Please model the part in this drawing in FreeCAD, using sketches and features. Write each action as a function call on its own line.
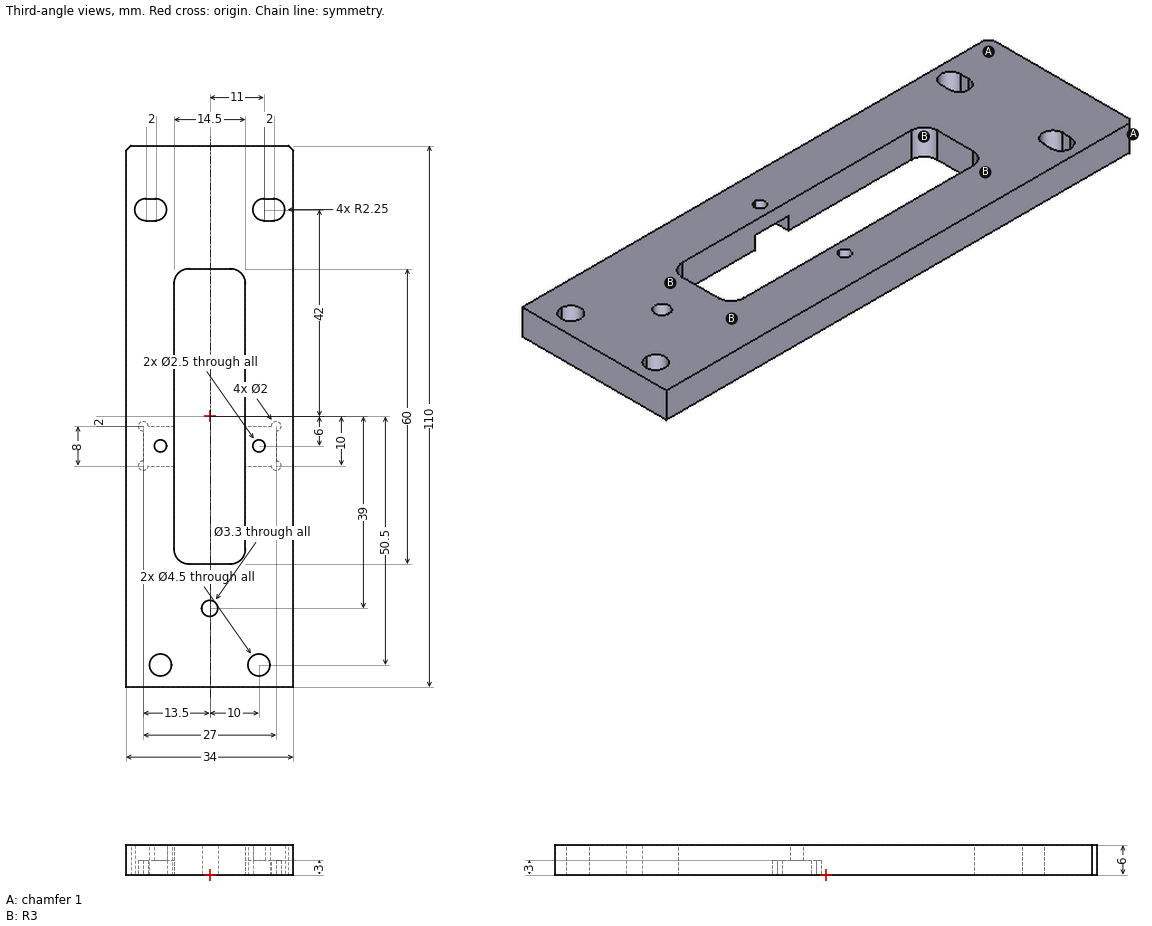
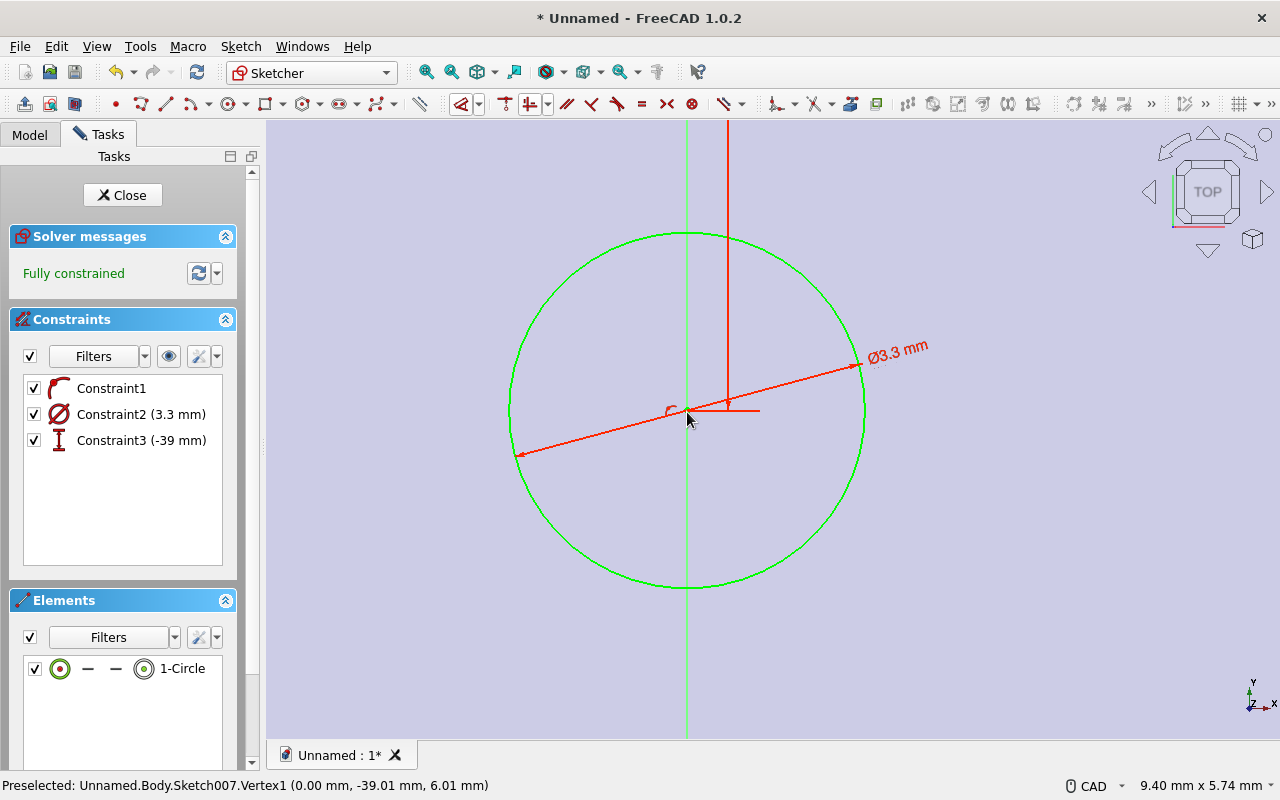
click(123, 195)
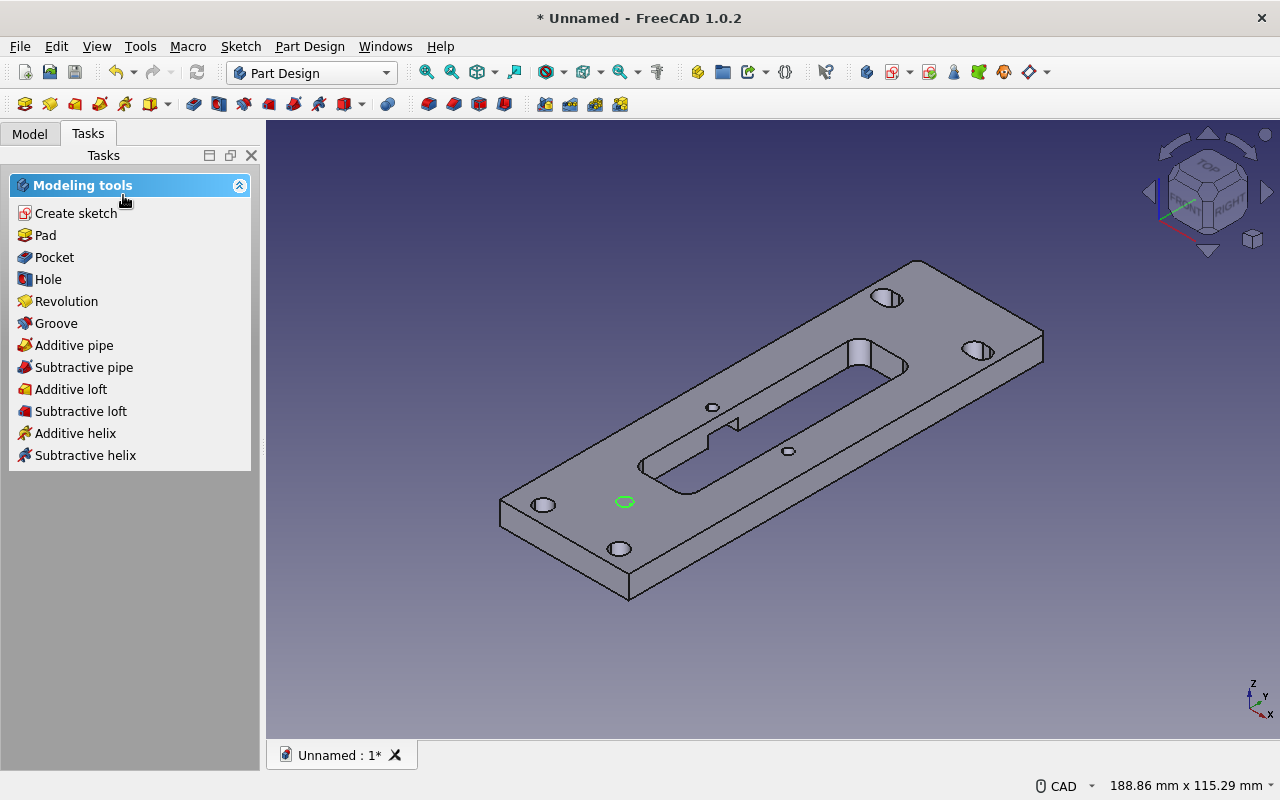
click(219, 104)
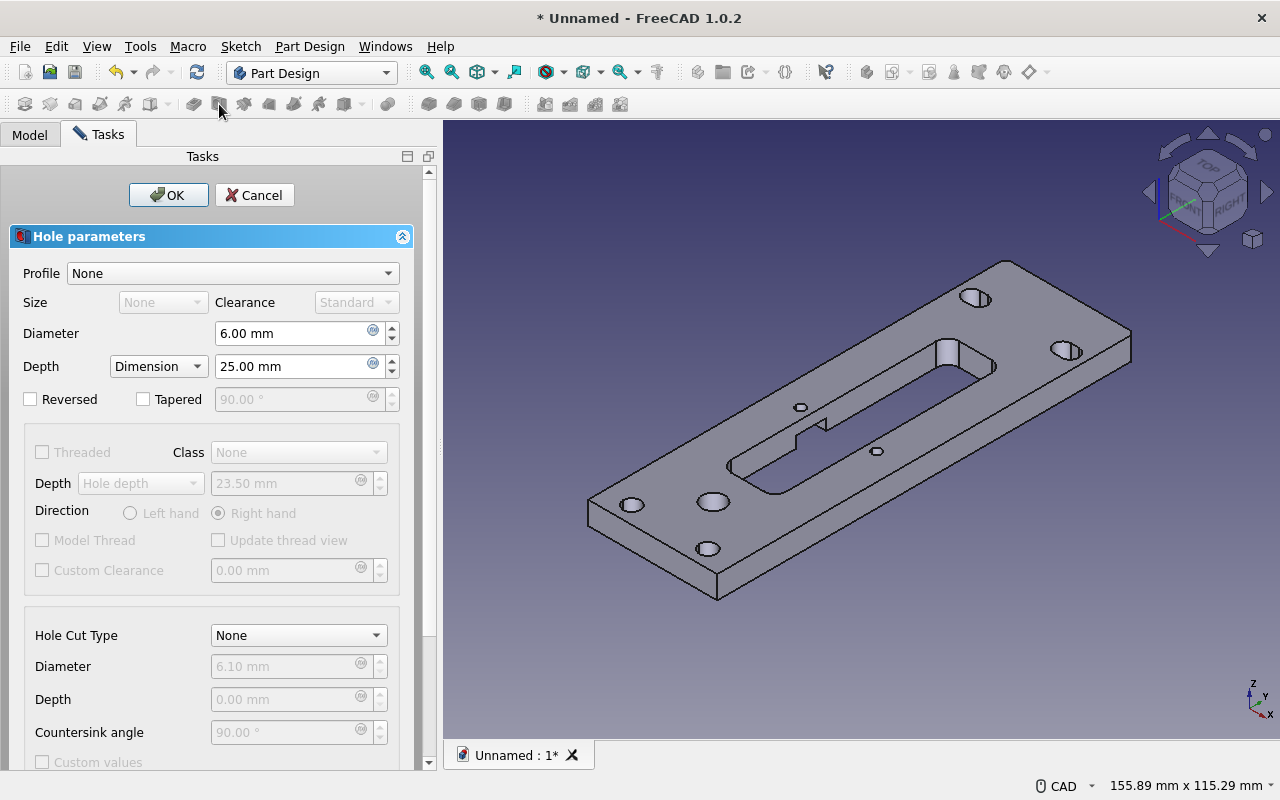
triple_click(300, 334)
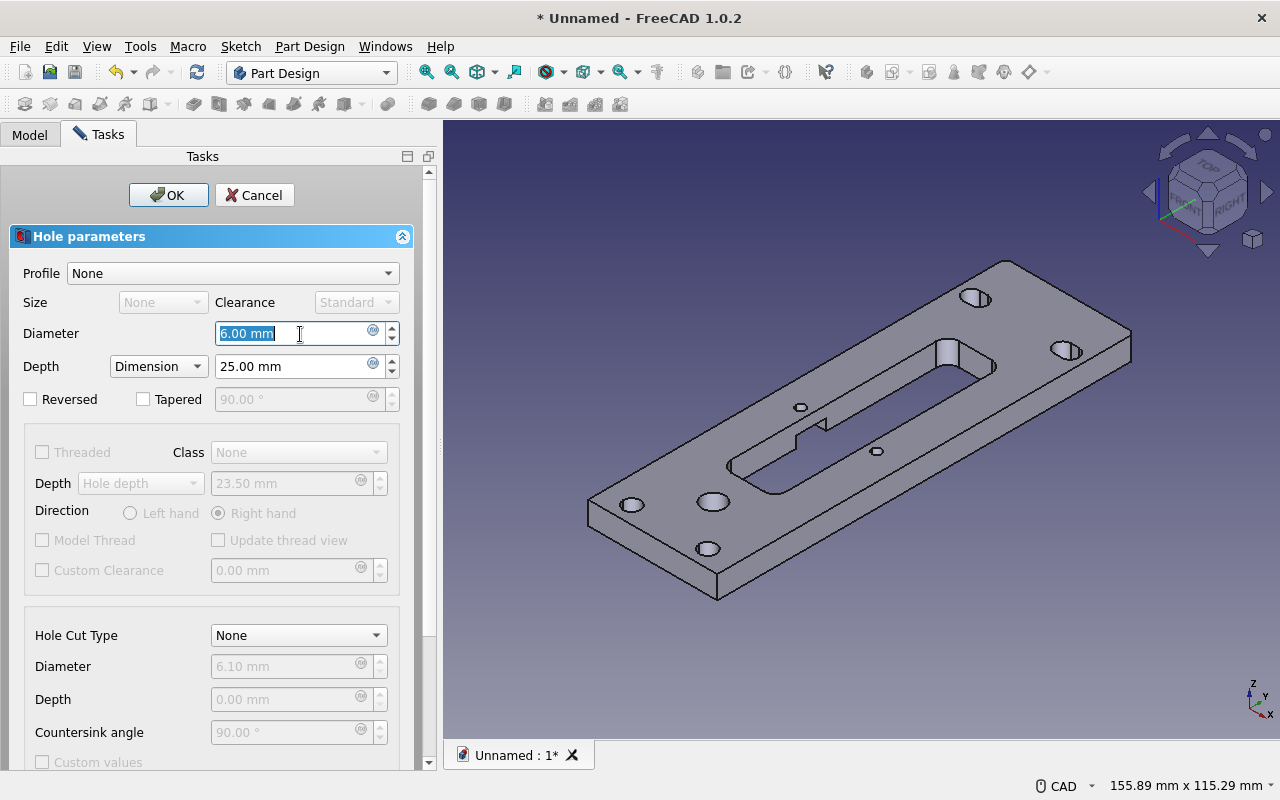
text(3.3)
key(Tab)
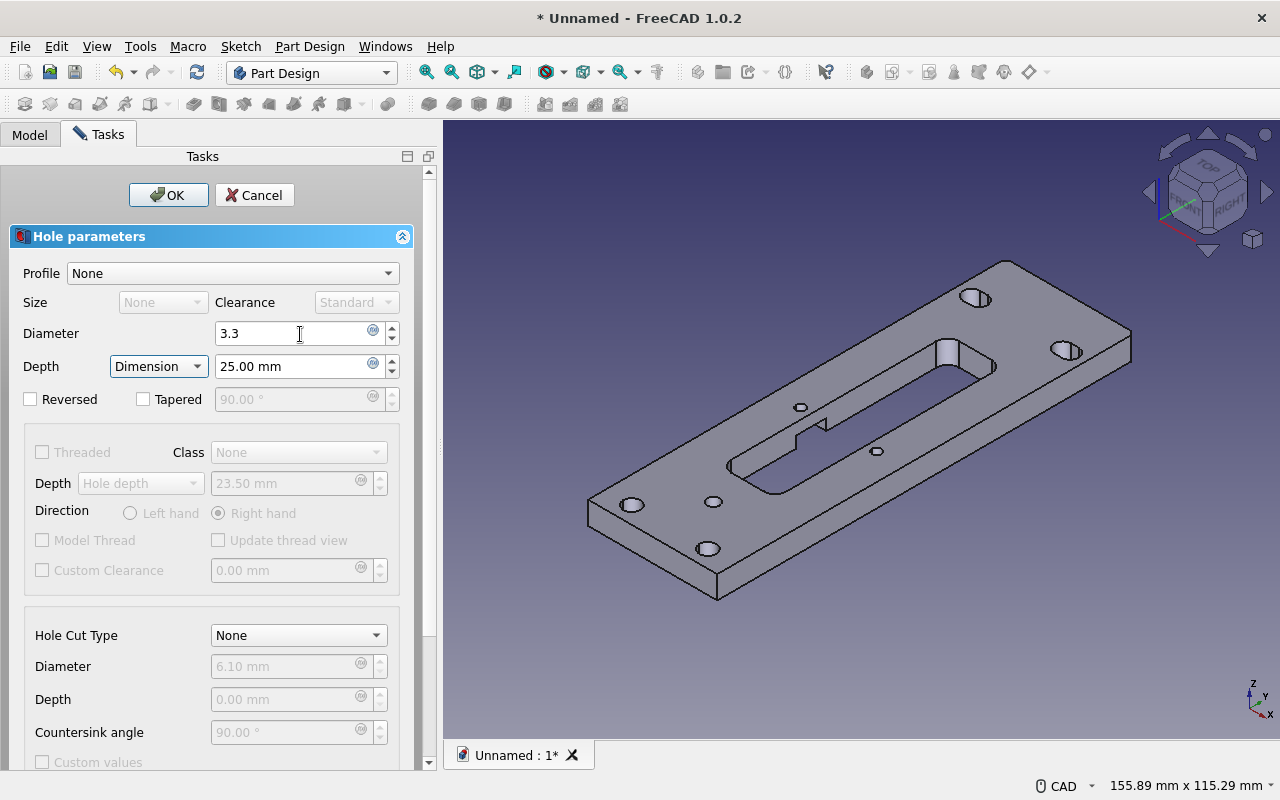
click(160, 366)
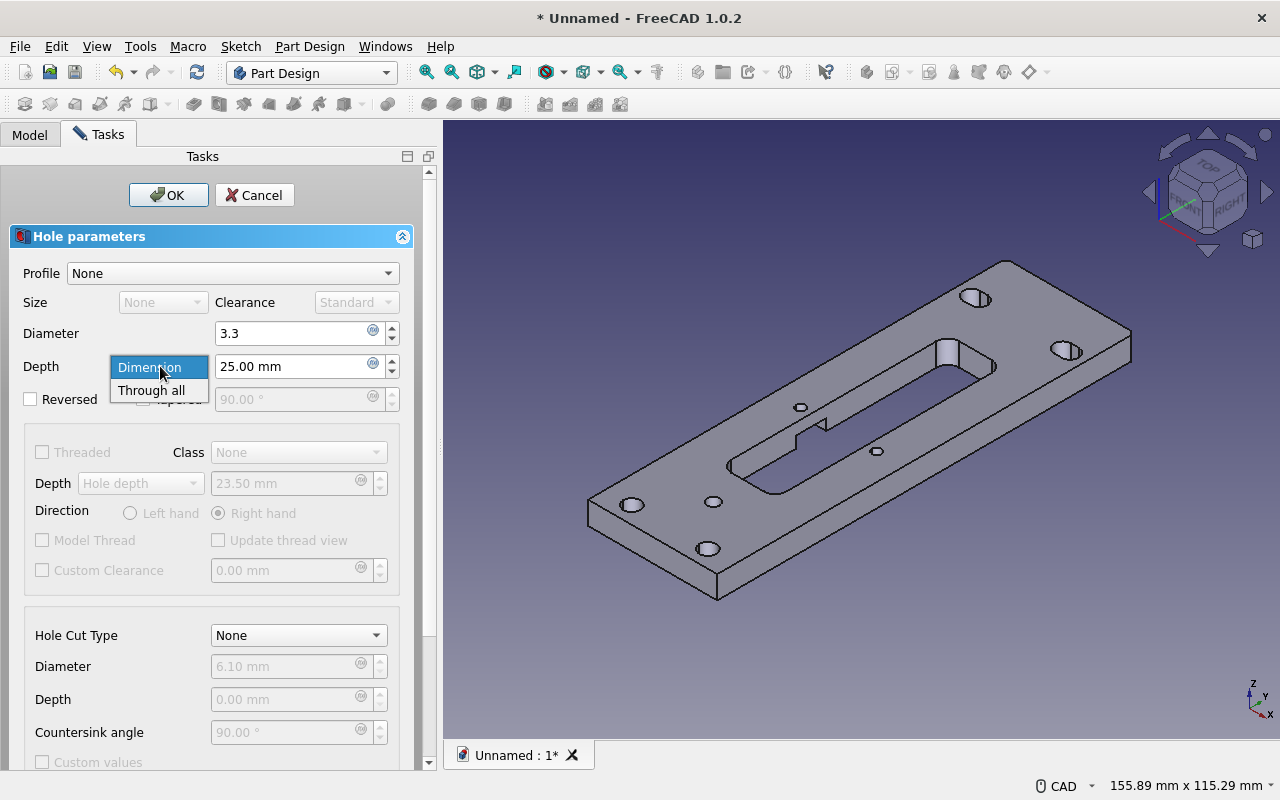
click(158, 390)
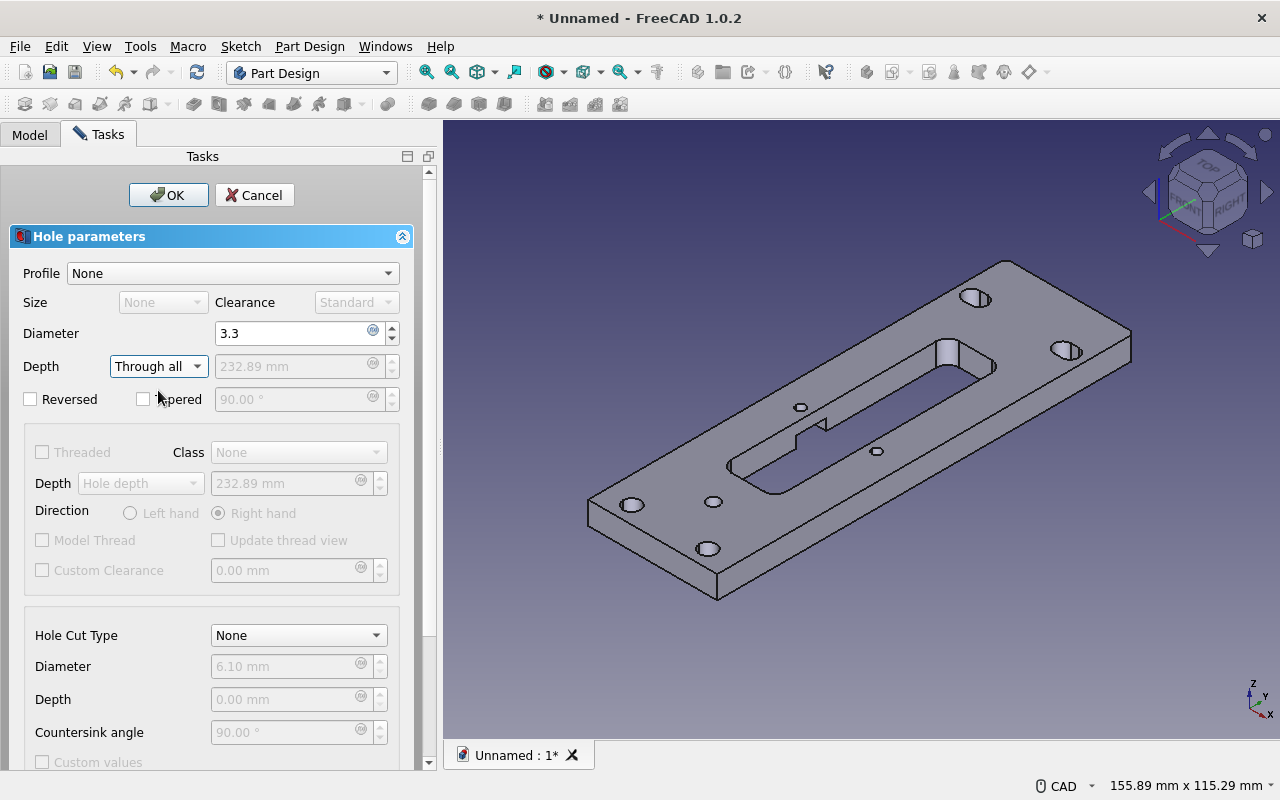
click(169, 195)